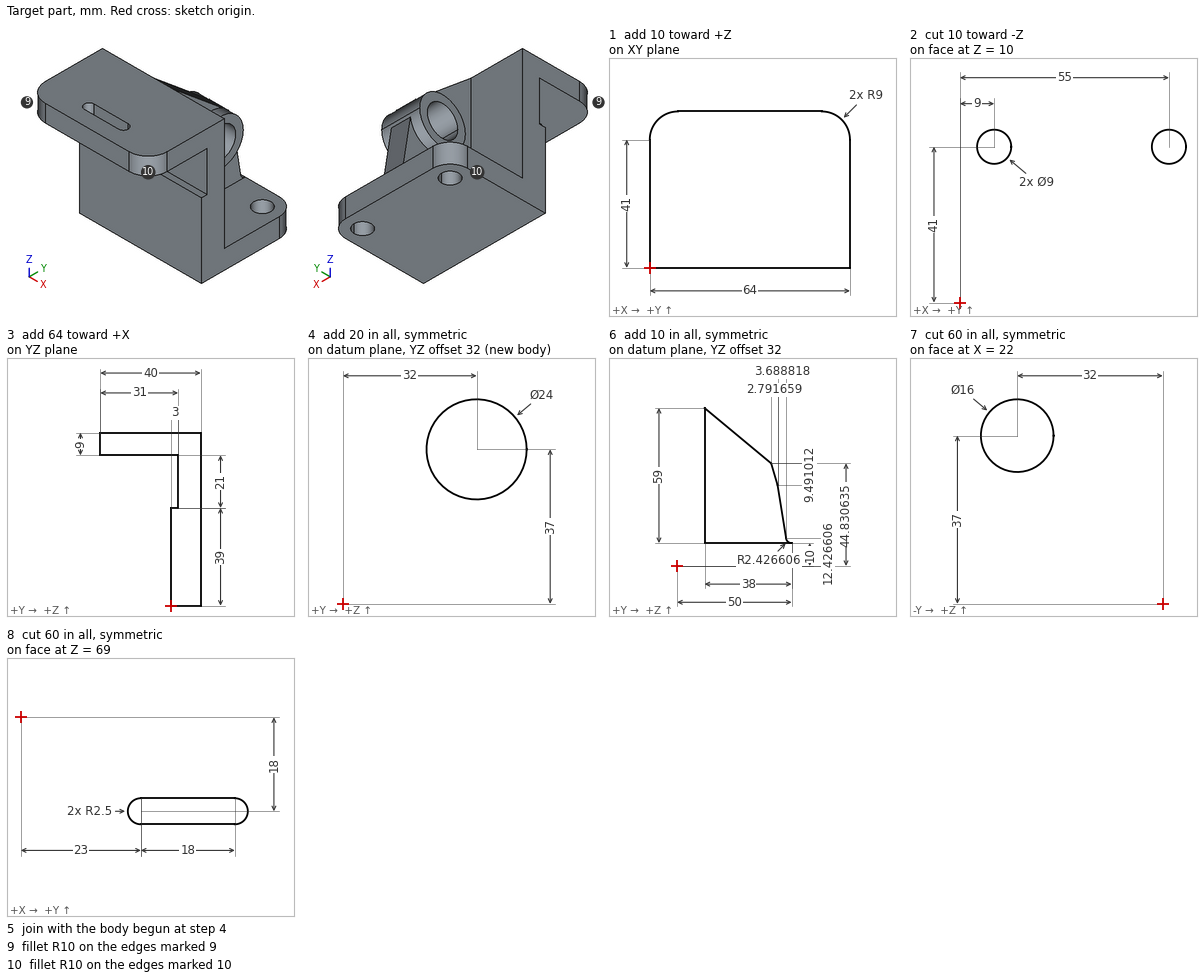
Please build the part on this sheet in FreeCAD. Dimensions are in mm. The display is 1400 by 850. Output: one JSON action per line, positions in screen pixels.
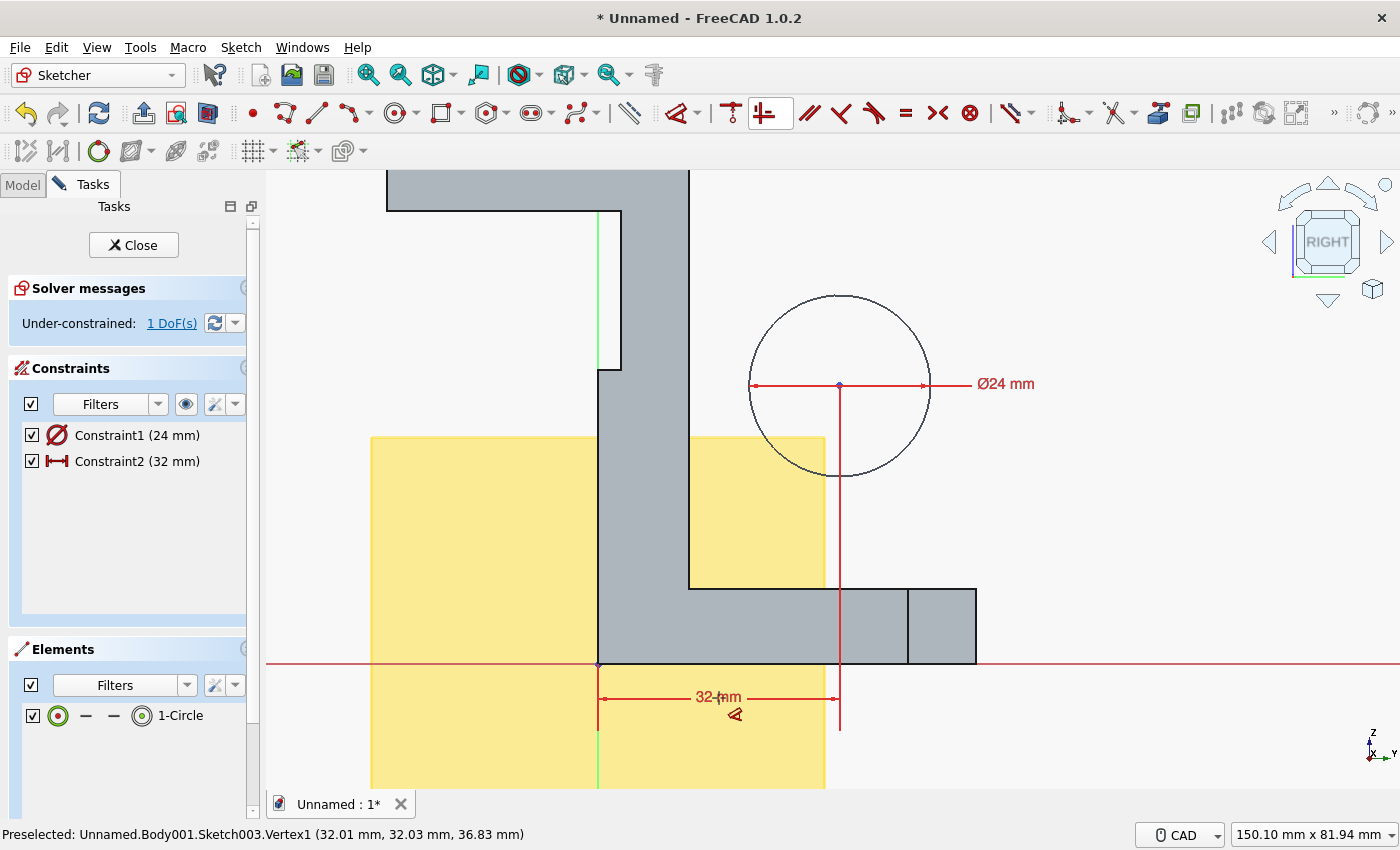
{"action": "left_click", "coordinate": [840, 386]}
{"action": "left_click", "coordinate": [564, 525]}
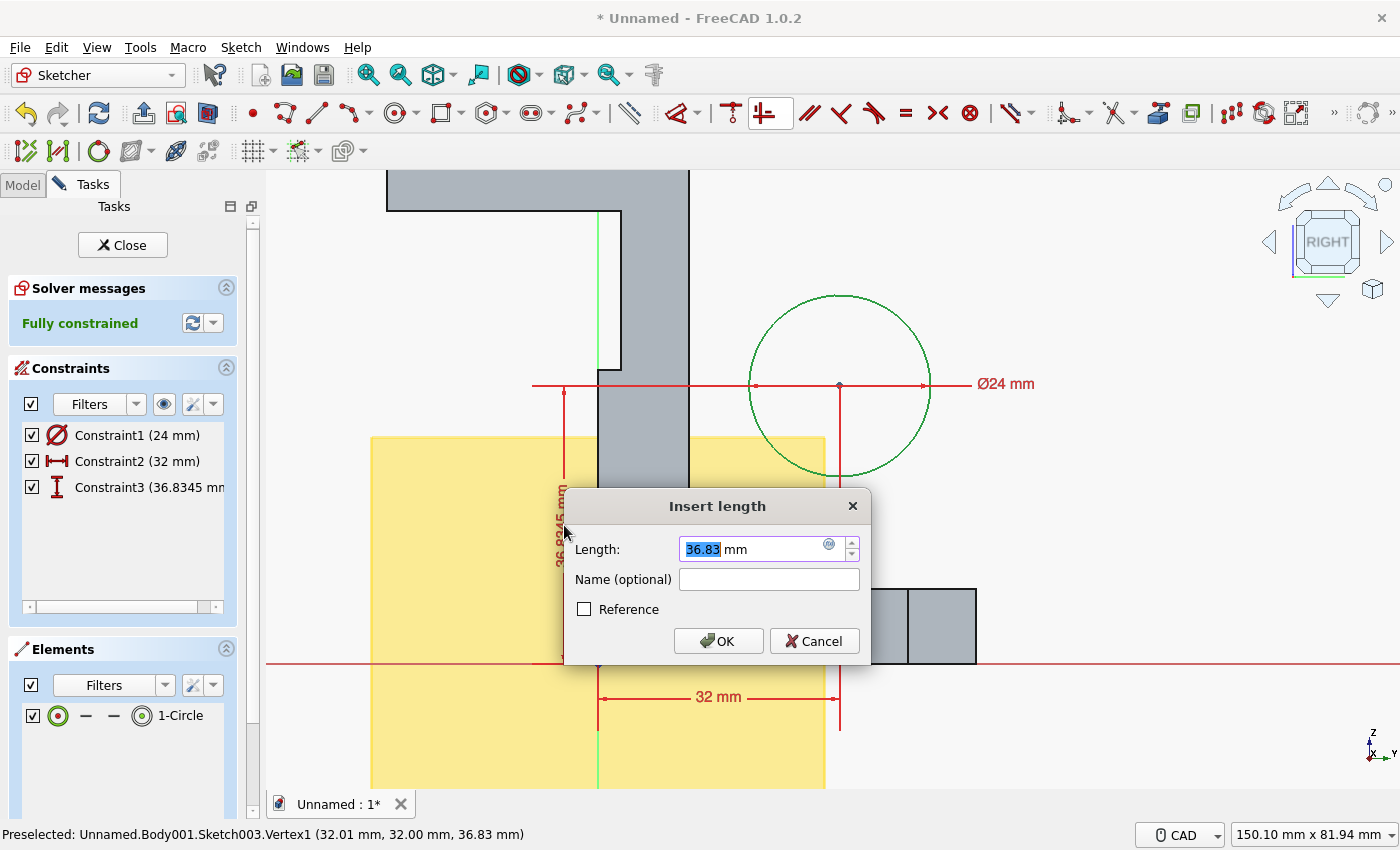
{"action": "type", "text": "37"}
{"action": "key", "text": "Return"}
{"action": "key", "text": "Escape"}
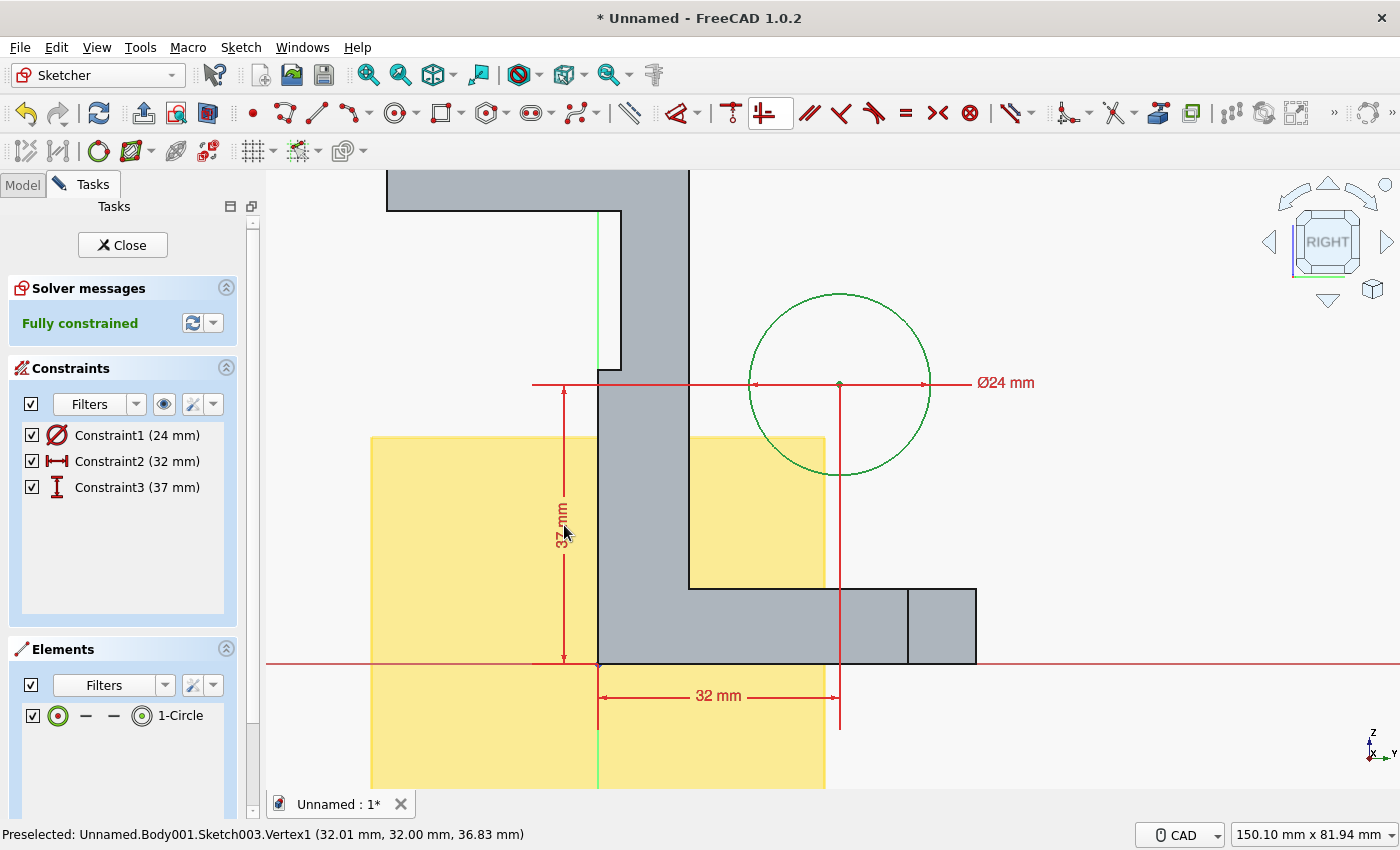
{"action": "left_click", "coordinate": [123, 245]}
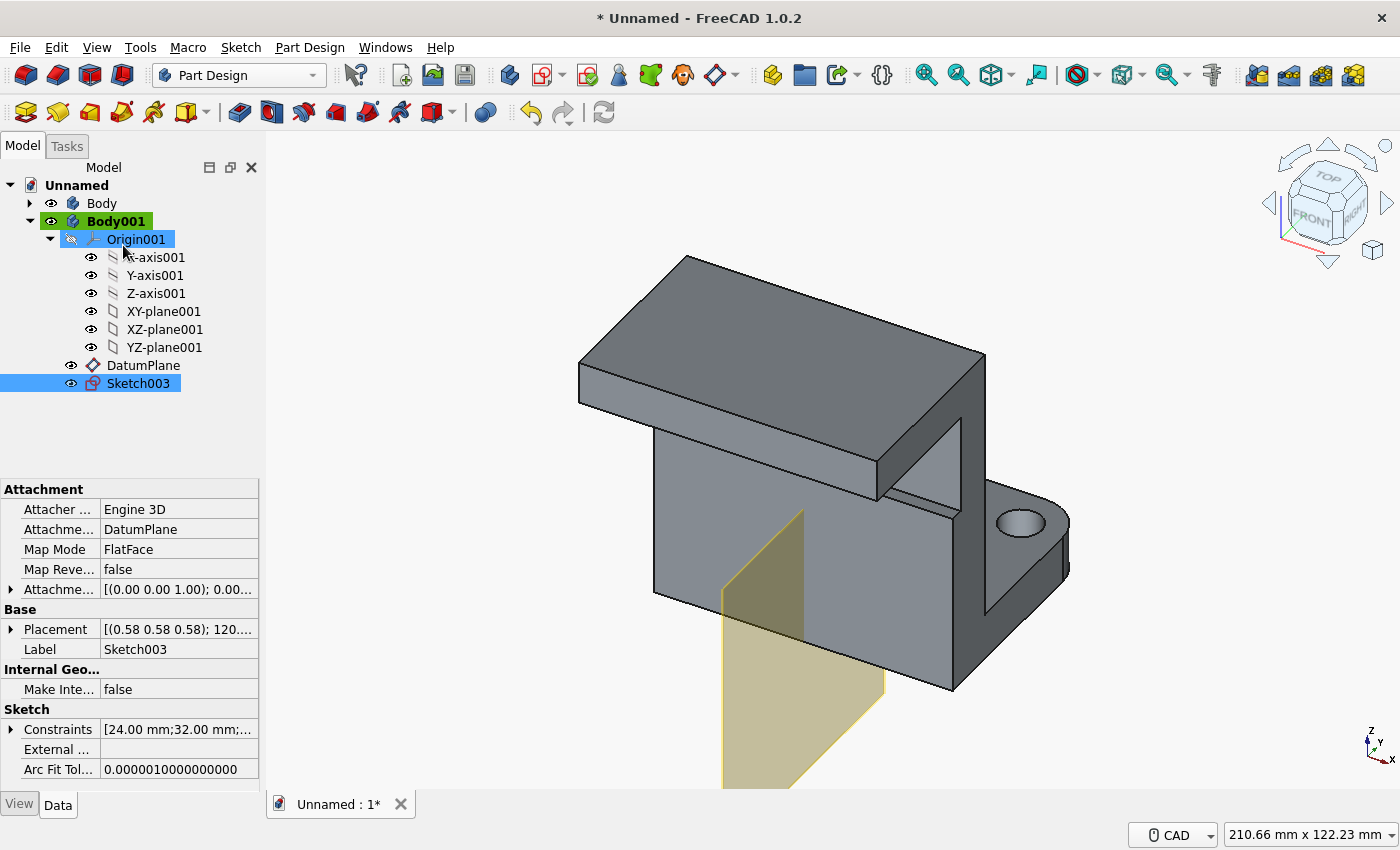
{"action": "left_click", "coordinate": [26, 112]}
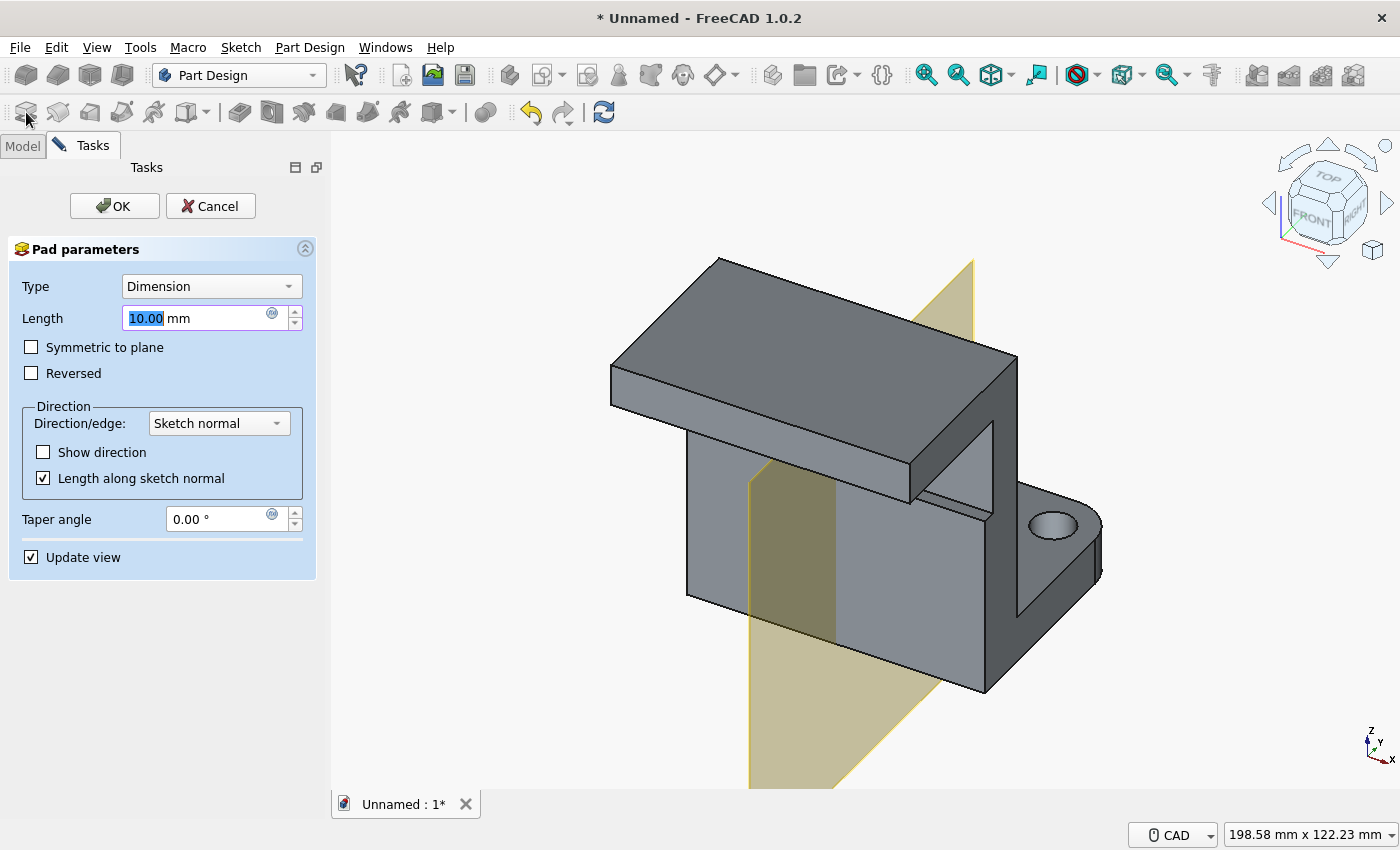
{"action": "type", "text": "20"}
{"action": "key", "text": "Tab"}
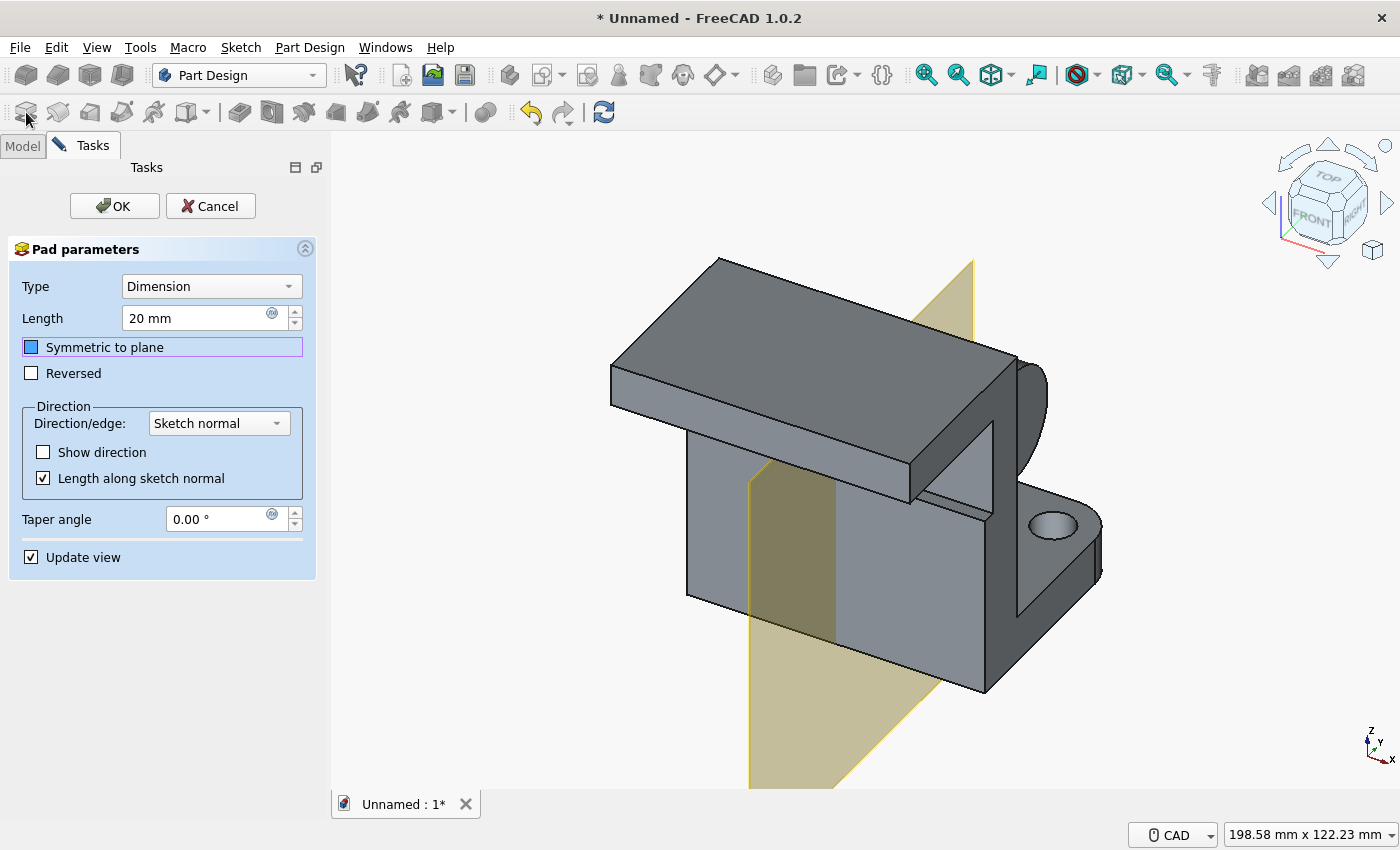
{"action": "left_click", "coordinate": [30, 347]}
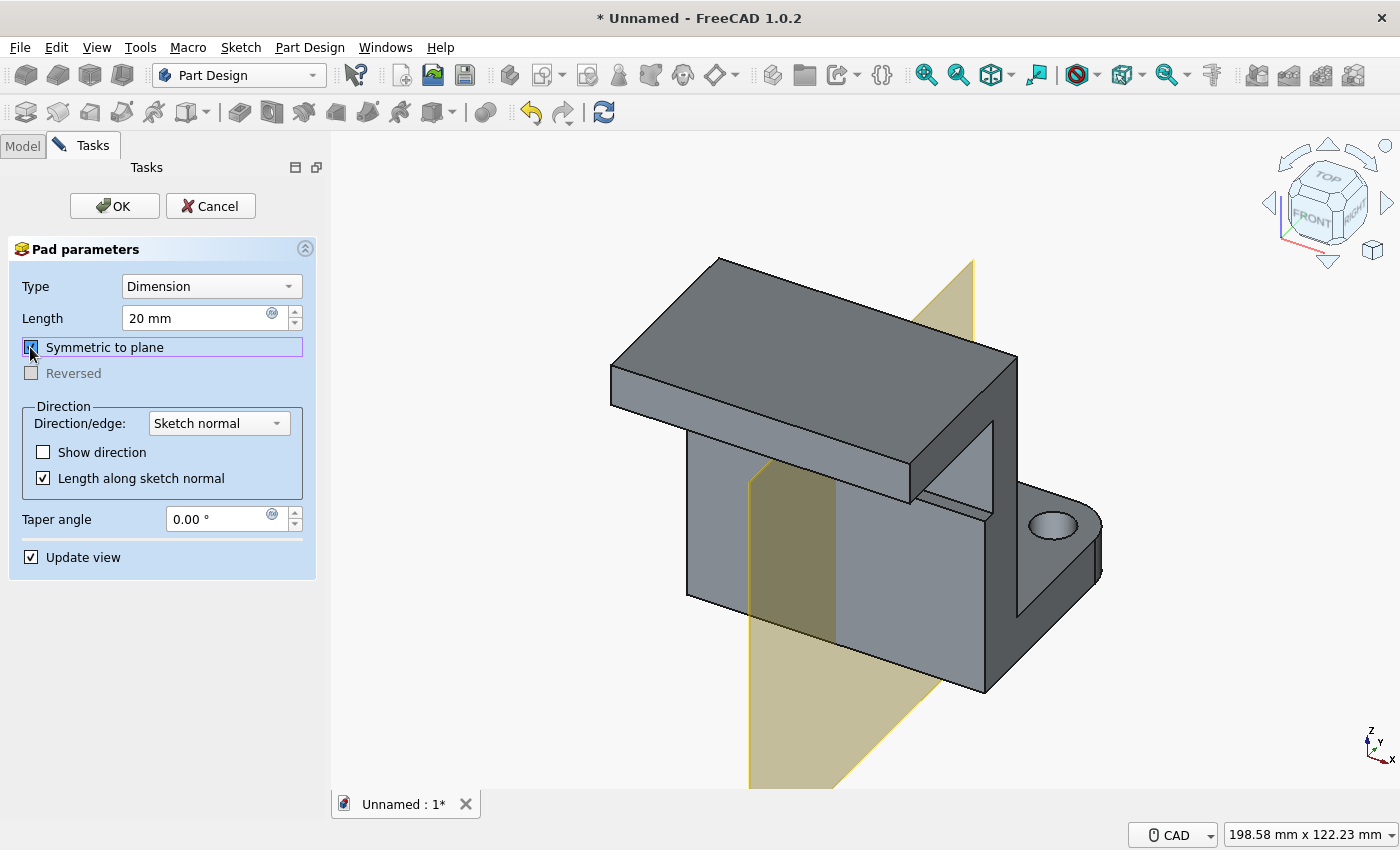
{"action": "left_click", "coordinate": [115, 206]}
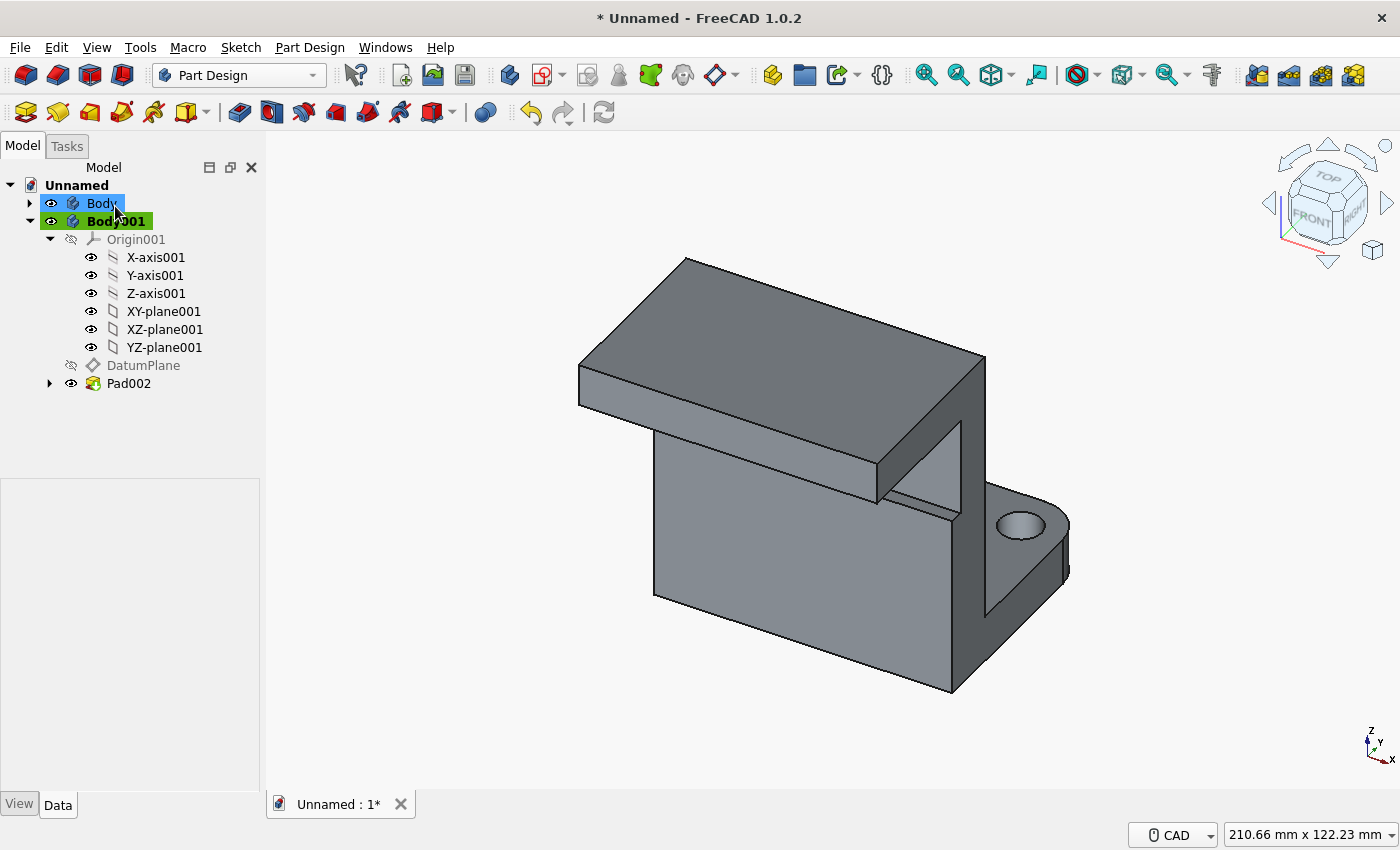
{"action": "left_click", "coordinate": [928, 76]}